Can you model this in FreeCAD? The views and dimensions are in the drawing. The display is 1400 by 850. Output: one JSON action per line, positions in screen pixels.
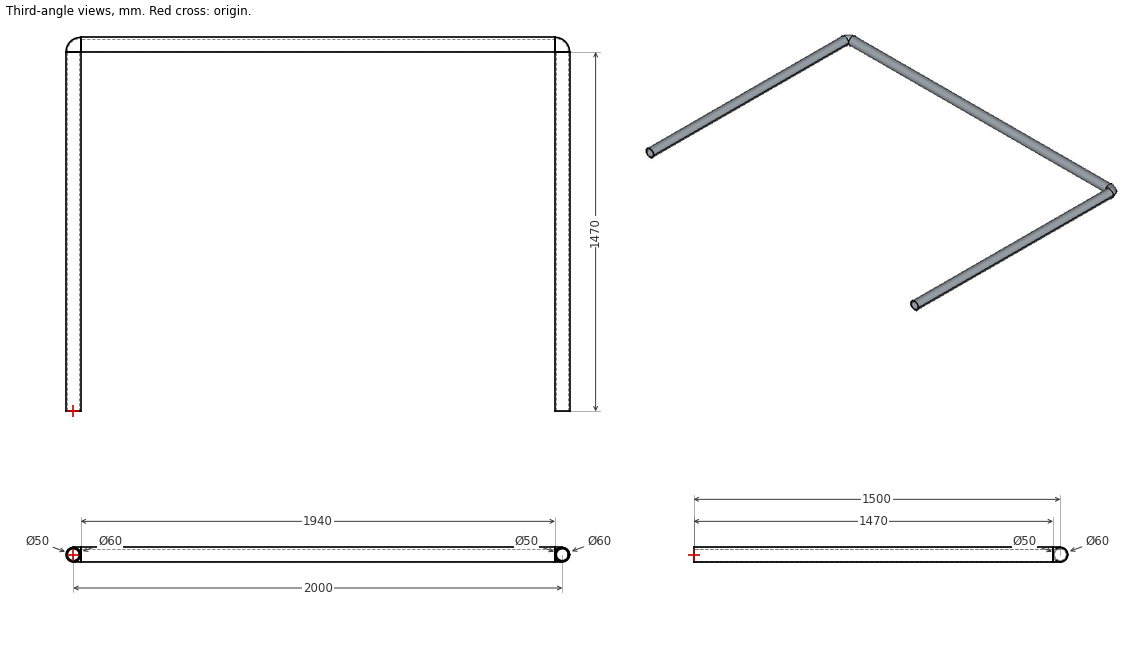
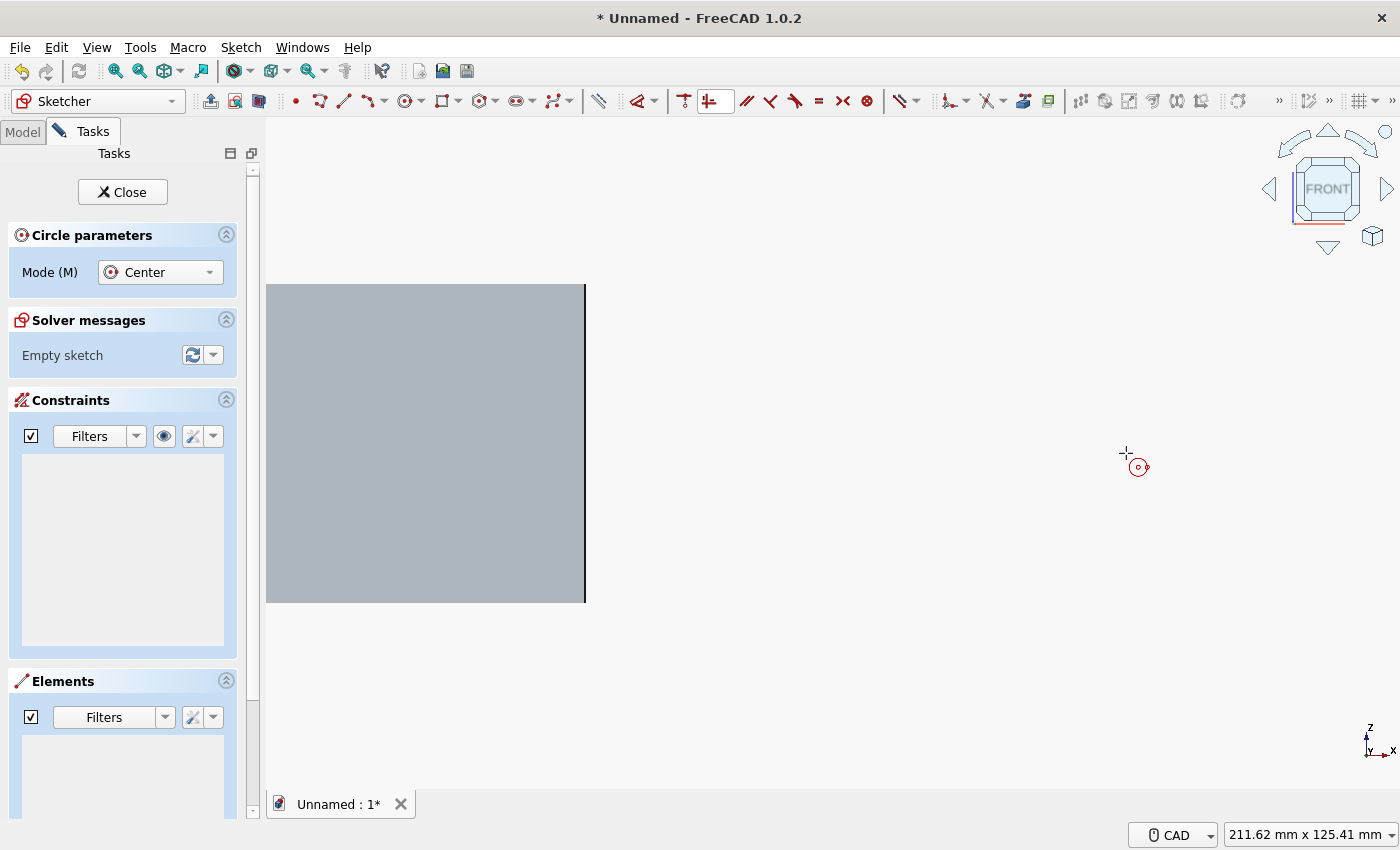
{"action": "left_click", "coordinate": [746, 443]}
{"action": "mouse_move", "coordinate": [860, 330]}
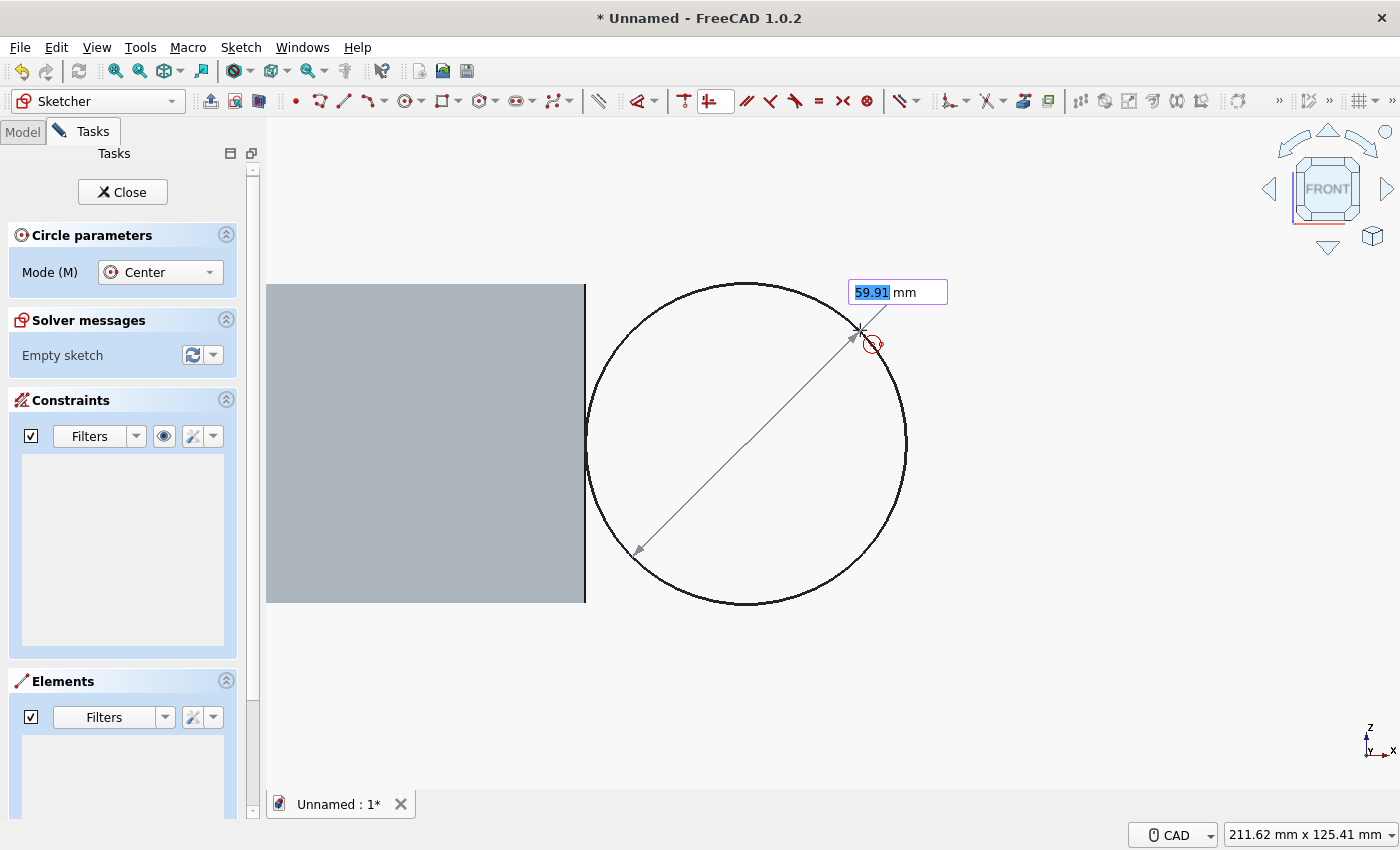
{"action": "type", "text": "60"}
{"action": "key", "text": "Return"}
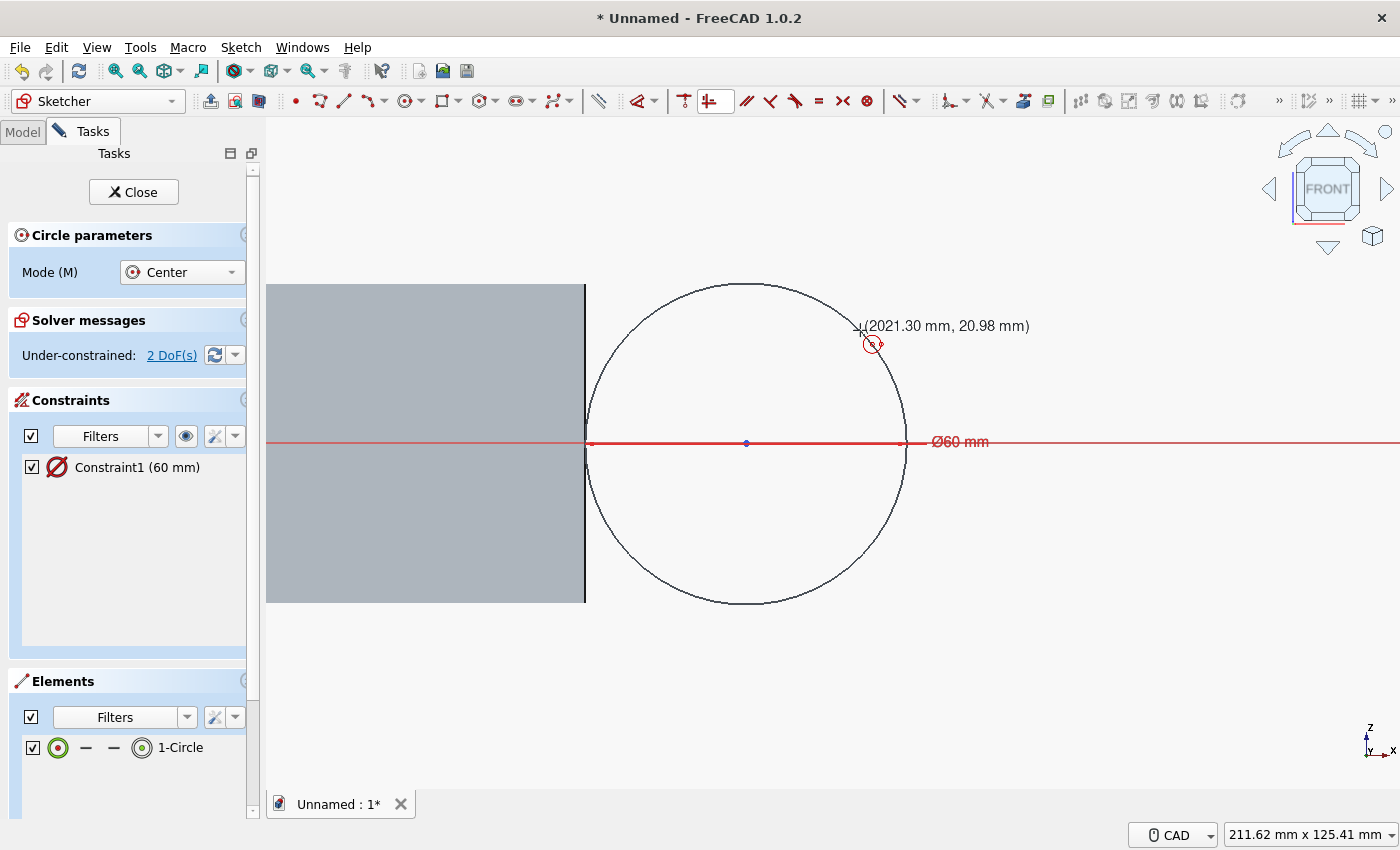
{"action": "left_click", "coordinate": [746, 444]}
{"action": "mouse_move", "coordinate": [841, 349]}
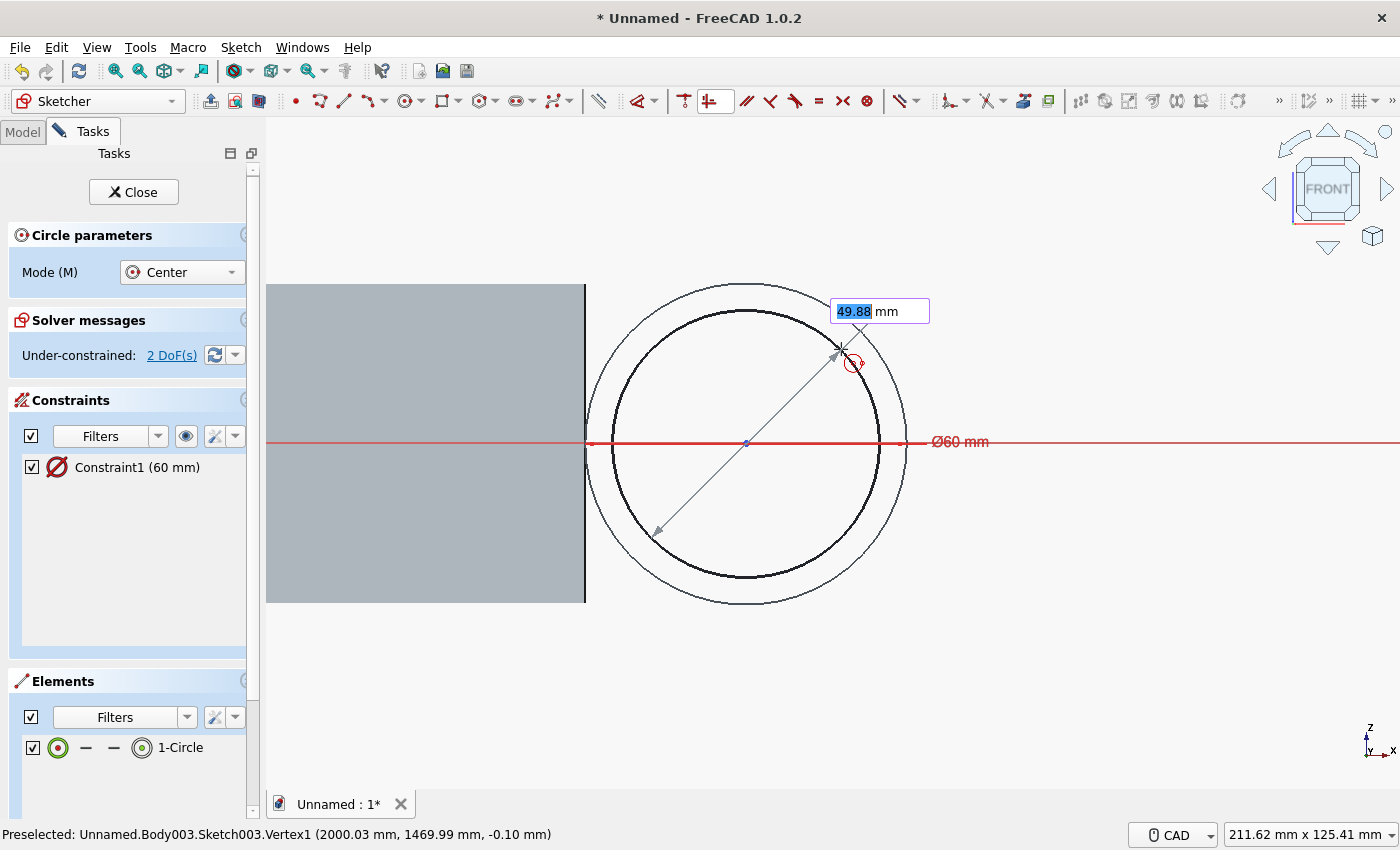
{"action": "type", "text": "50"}
{"action": "key", "text": "Return"}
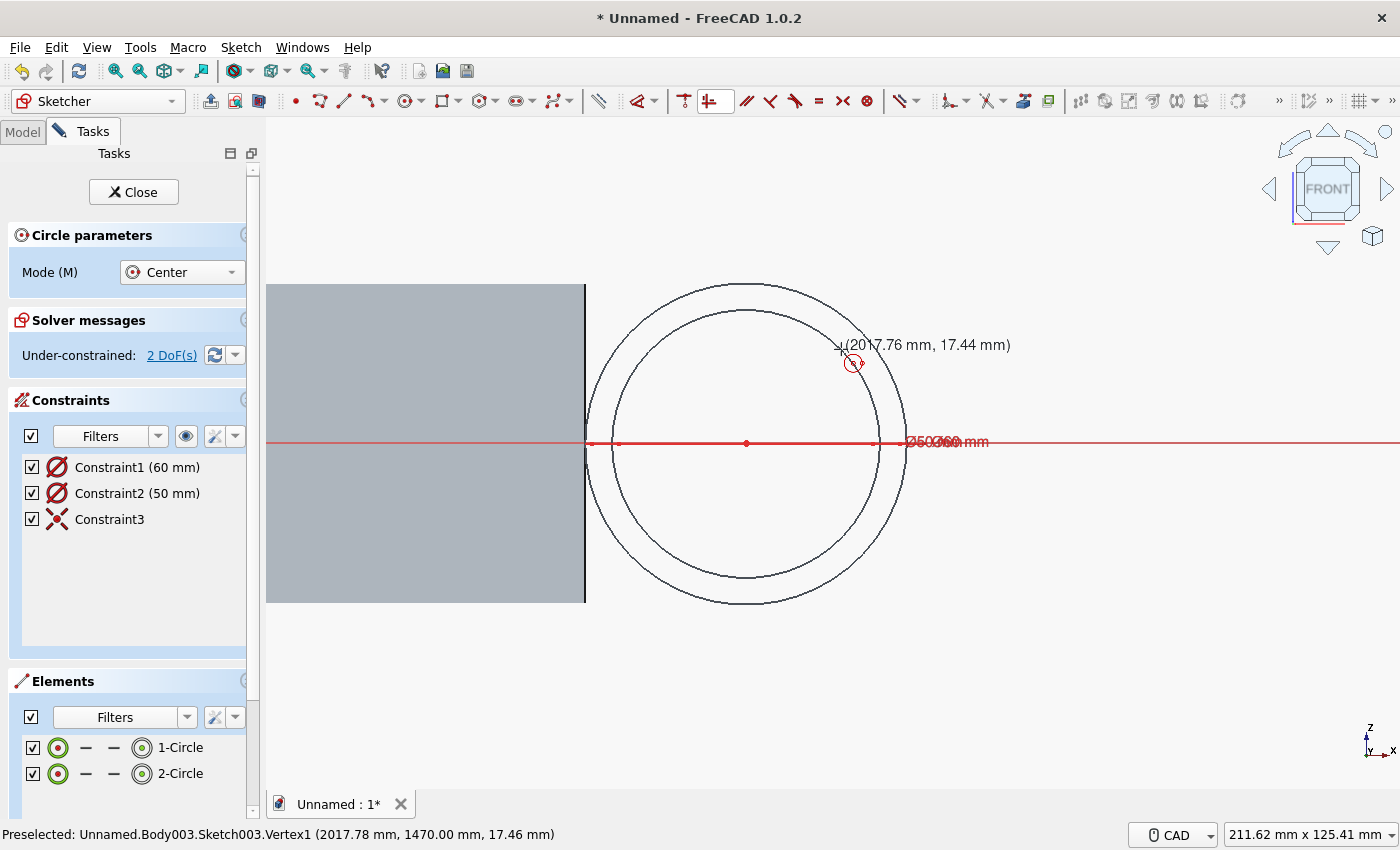
{"action": "left_click", "coordinate": [344, 102]}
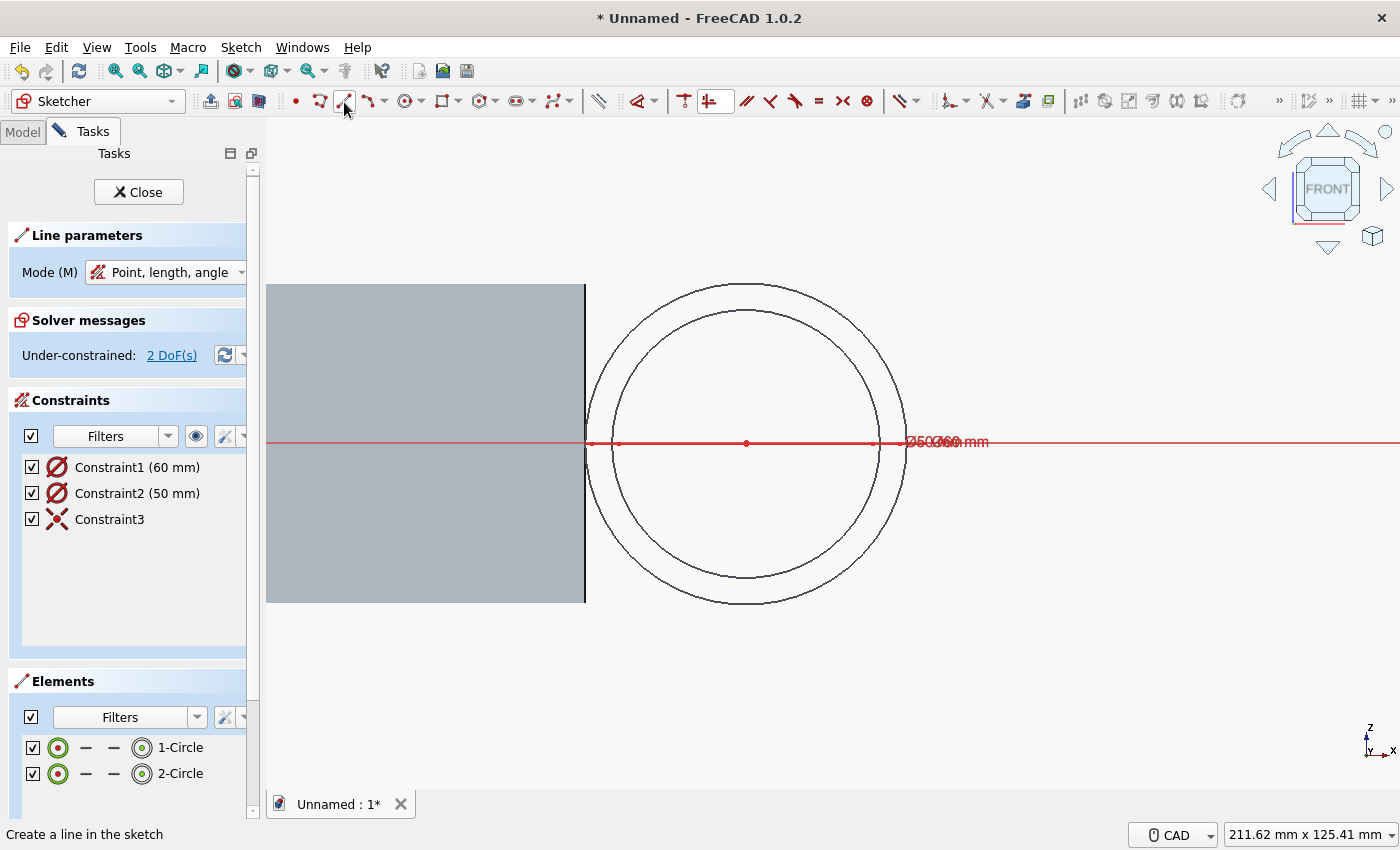
{"action": "left_click", "coordinate": [585, 636]}
{"action": "left_click", "coordinate": [585, 251]}
{"action": "key", "text": "Escape"}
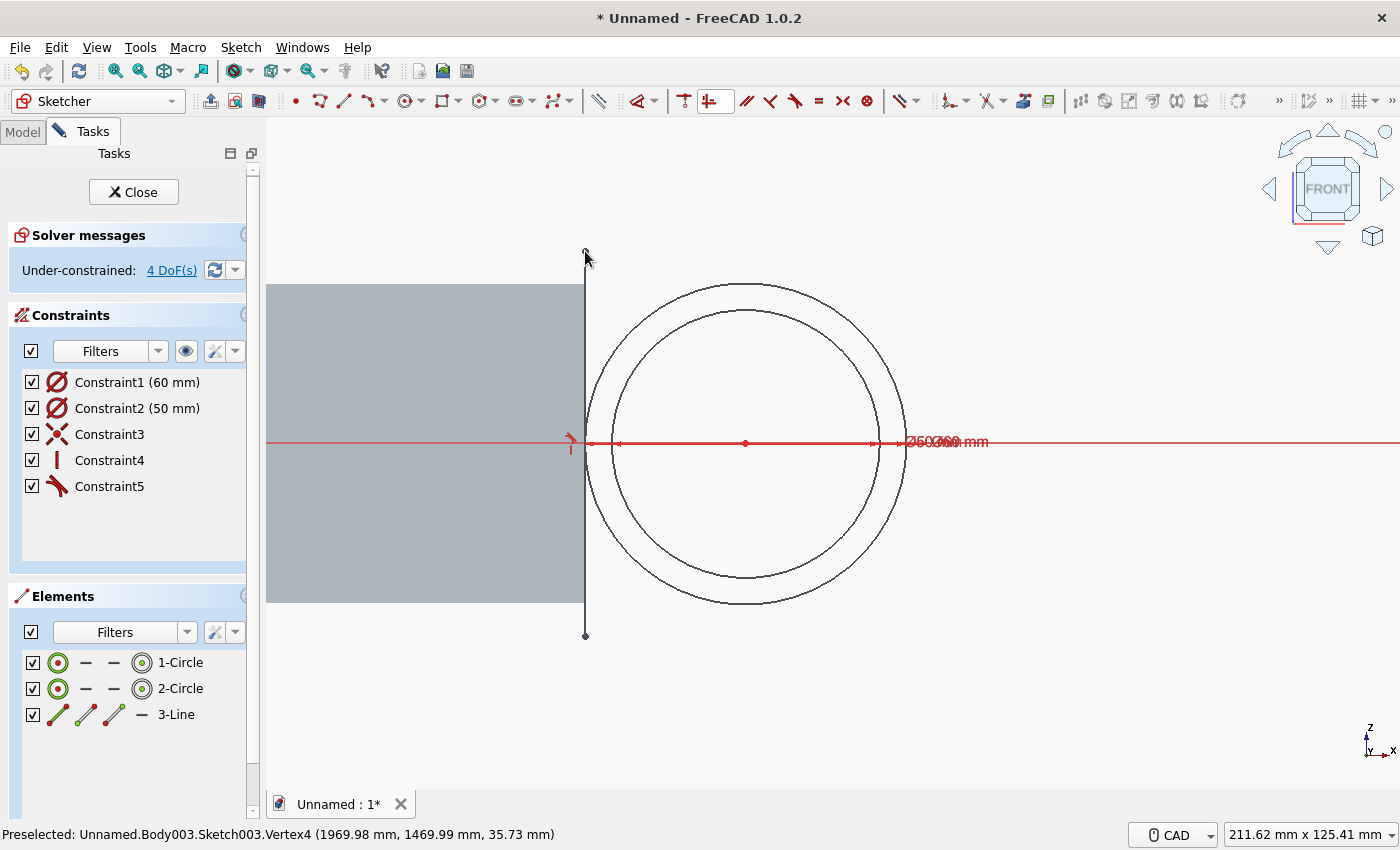
{"action": "left_click", "coordinate": [585, 521]}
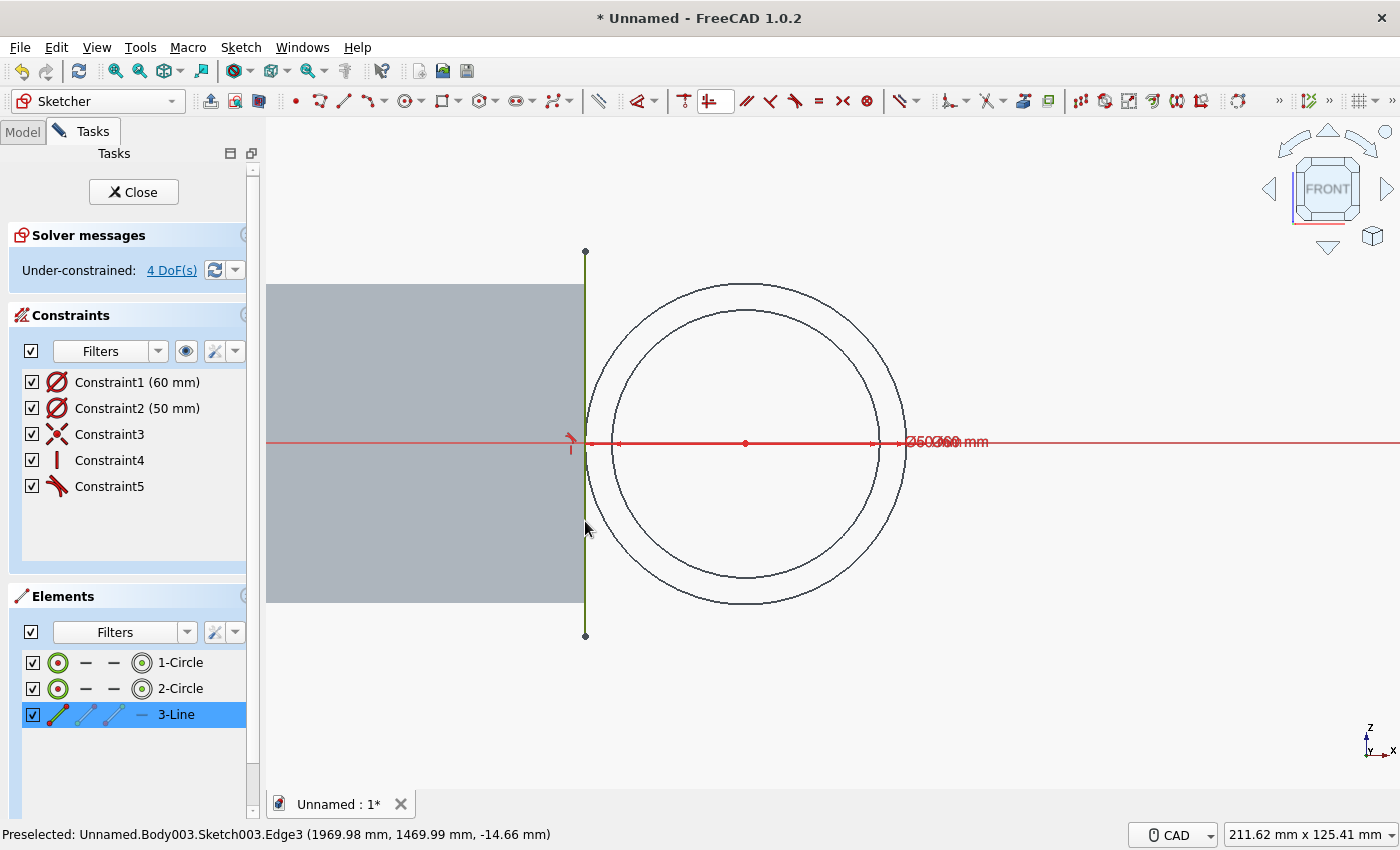
{"action": "key", "text": "g n"}